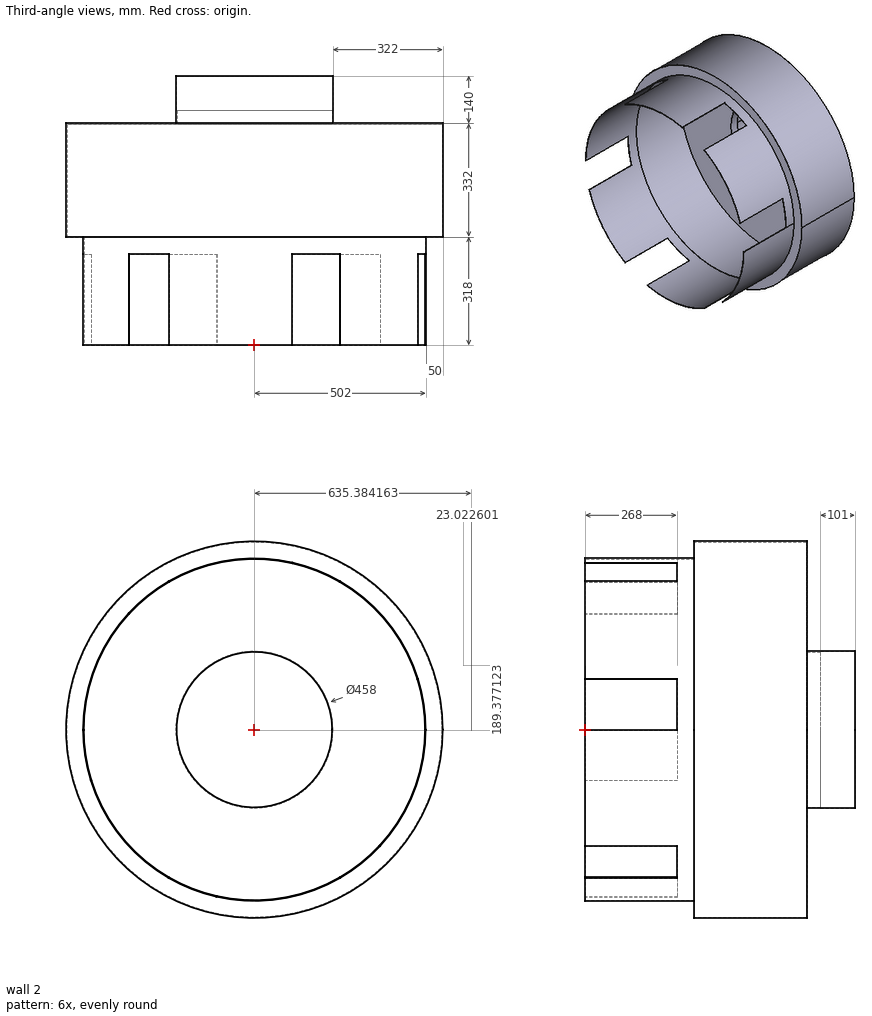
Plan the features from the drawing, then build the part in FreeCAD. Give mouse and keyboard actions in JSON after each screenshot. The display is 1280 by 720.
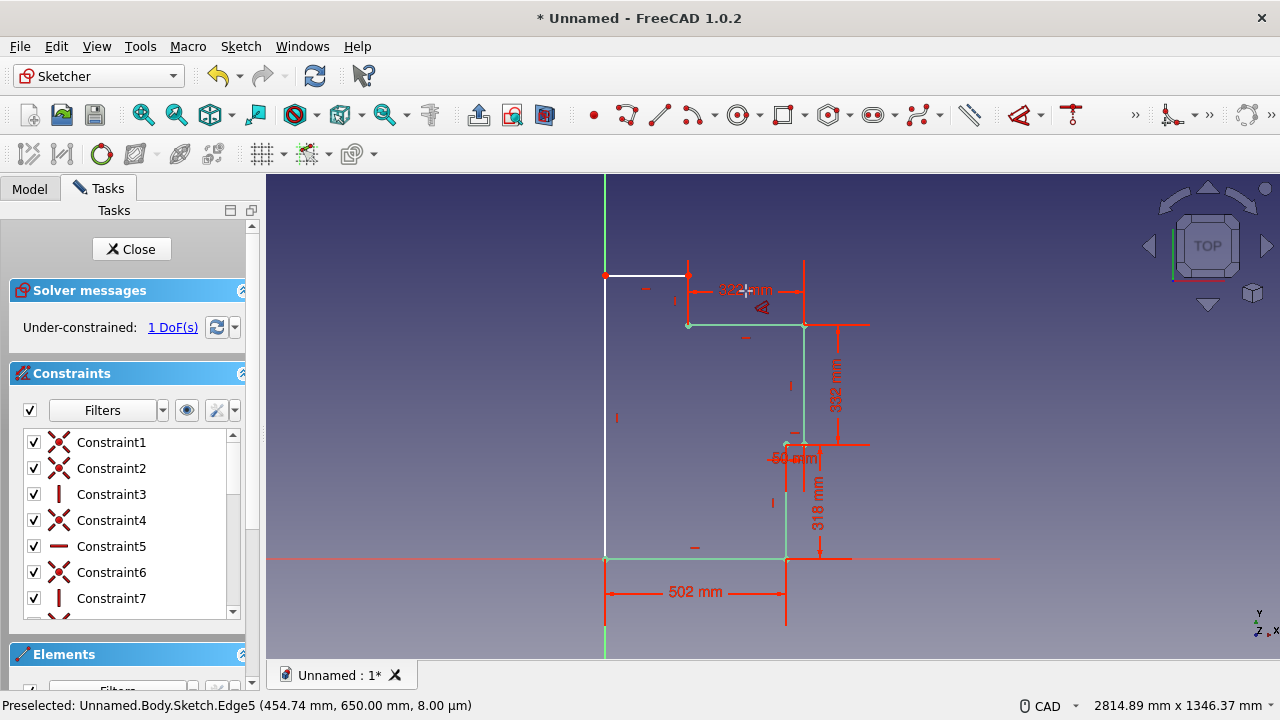
{"action": "left_click", "coordinate": [688, 310]}
{"action": "left_click", "coordinate": [654, 301]}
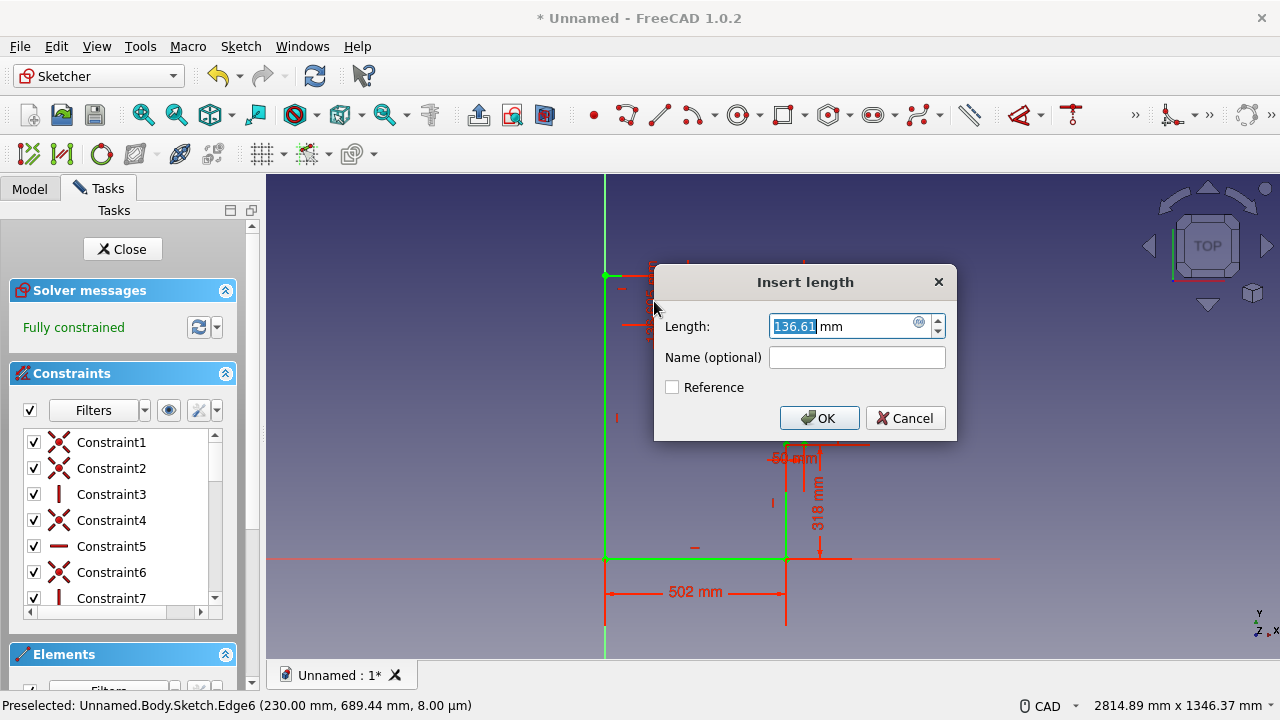
{"action": "type", "text": "140"}
{"action": "key", "text": "Return"}
{"action": "key", "text": "Escape"}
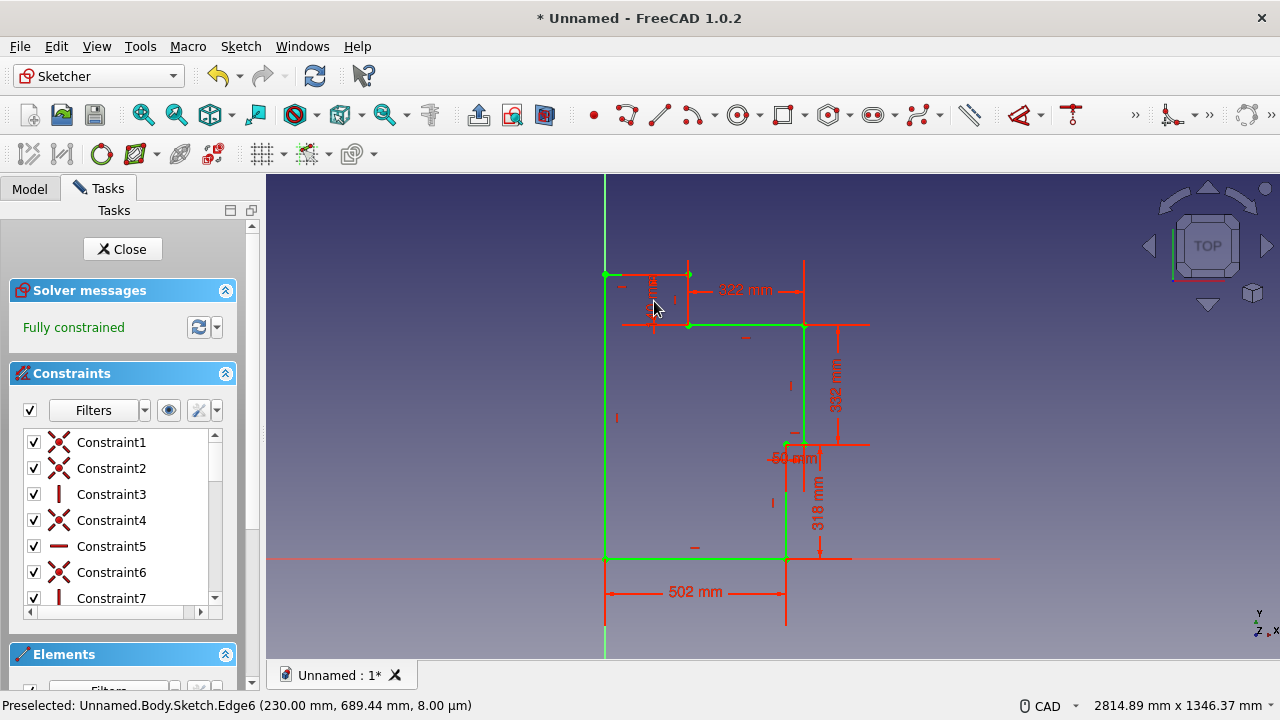
{"action": "left_click", "coordinate": [123, 249]}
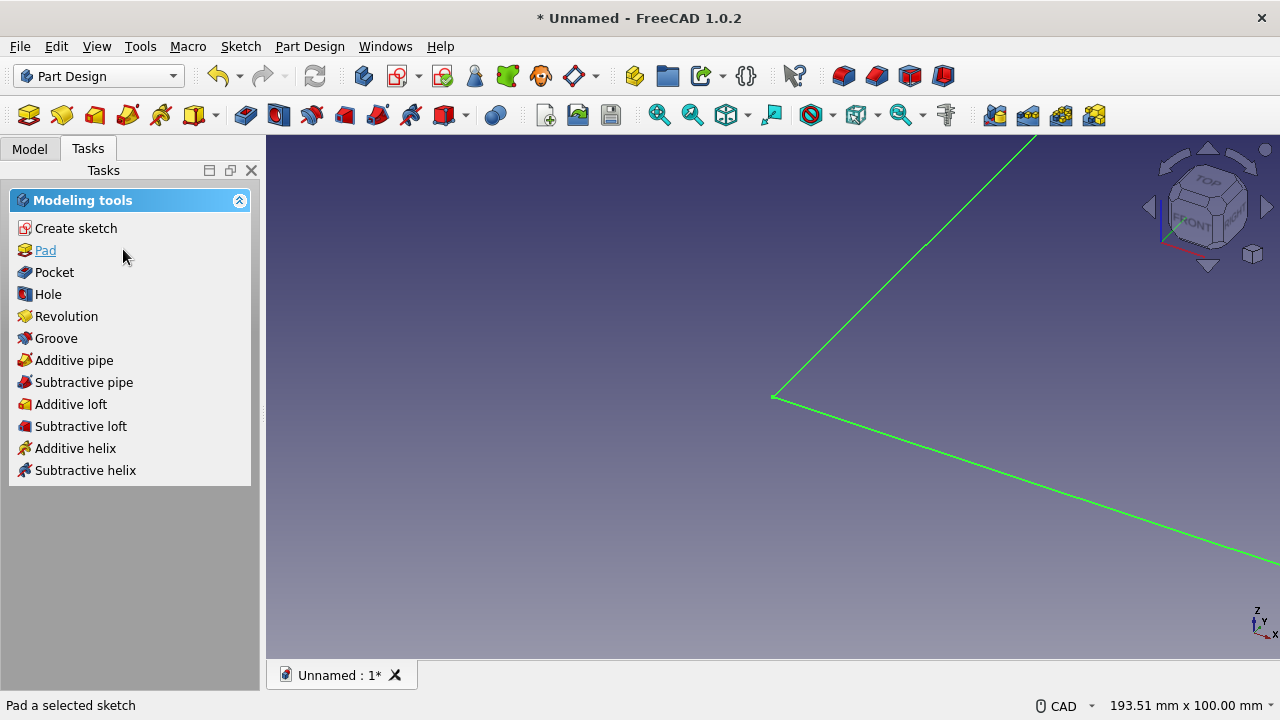
{"action": "left_click", "coordinate": [62, 116]}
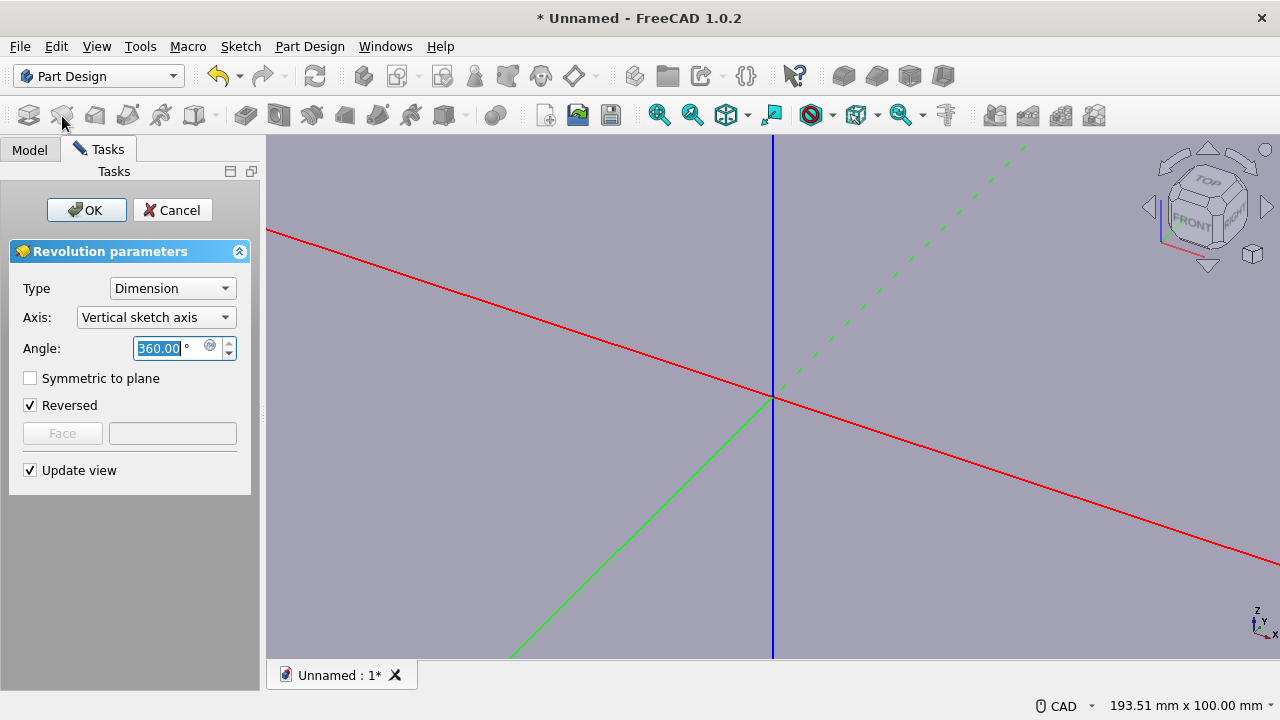
{"action": "left_click", "coordinate": [87, 210]}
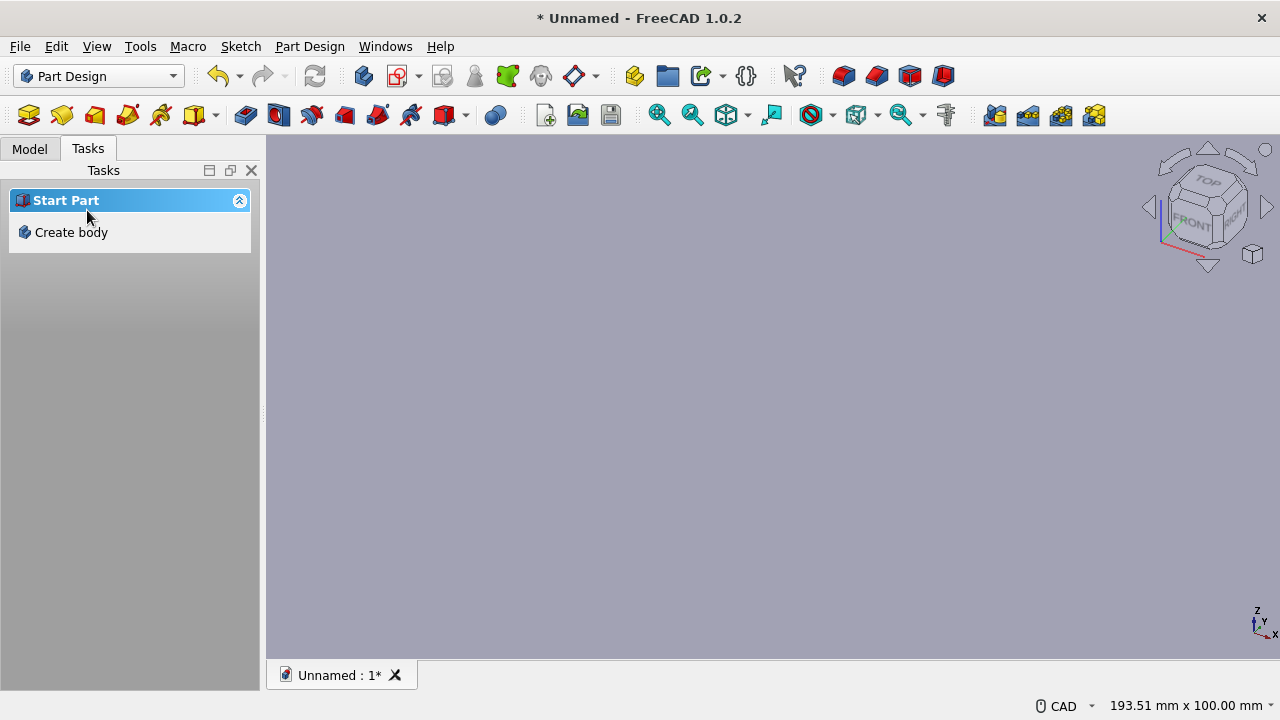
{"action": "left_click", "coordinate": [660, 116]}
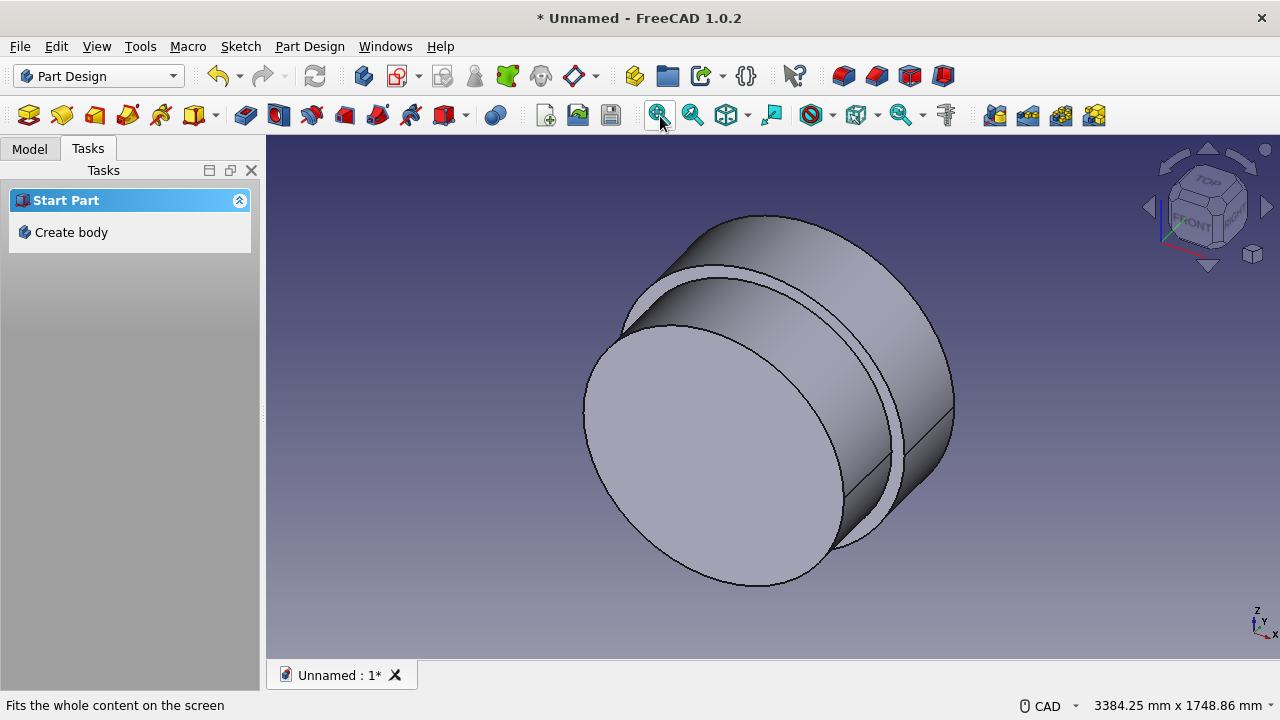
{"action": "left_click", "coordinate": [714, 455]}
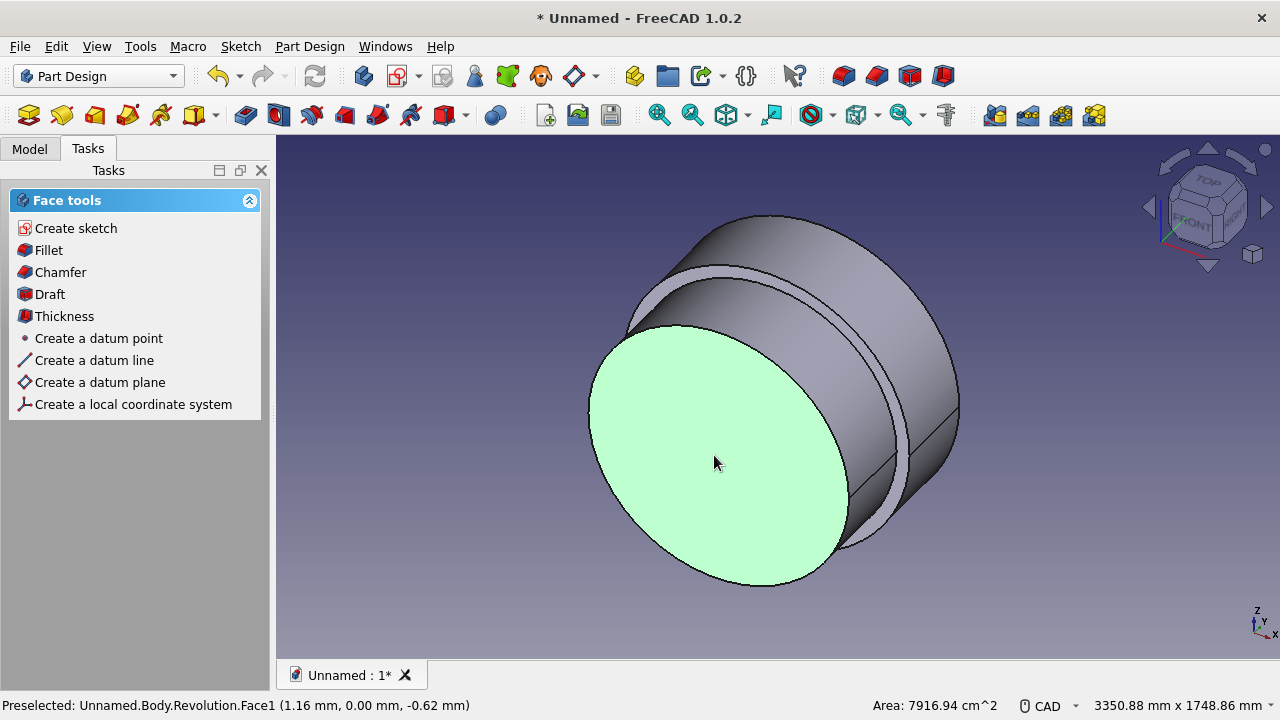
{"action": "left_click", "coordinate": [943, 76]}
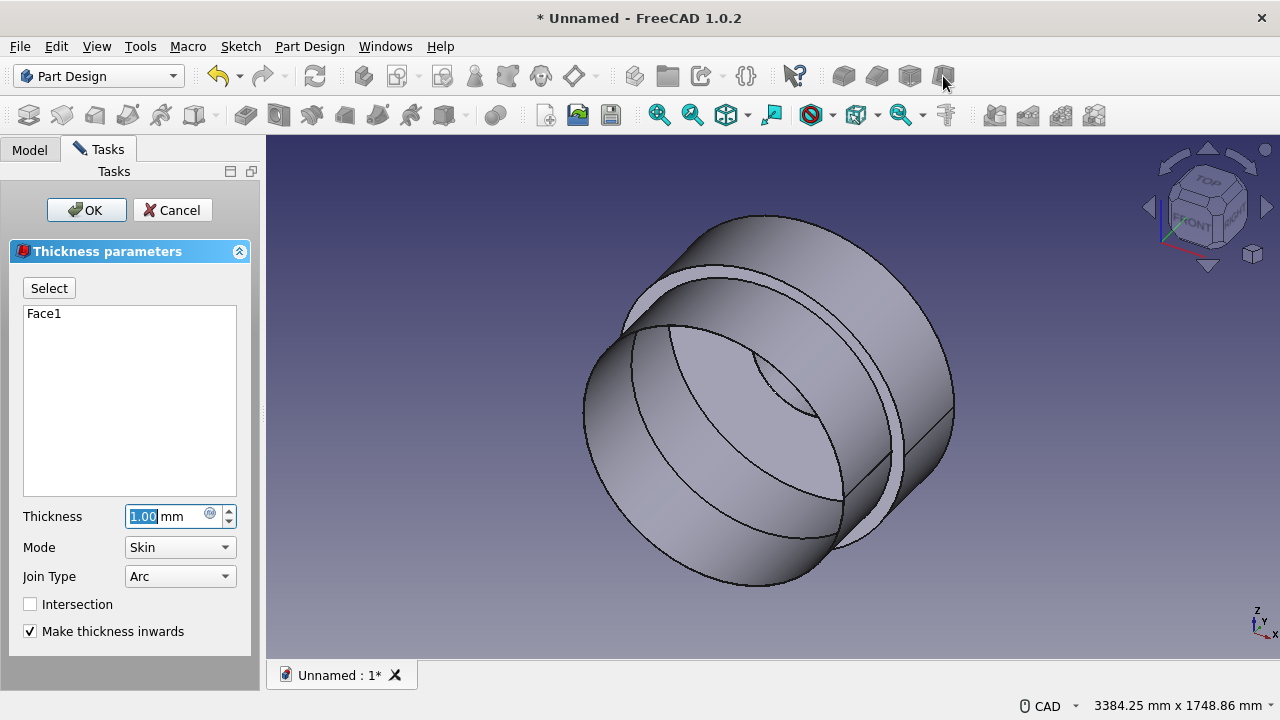
{"action": "type", "text": "2"}
{"action": "key", "text": "Tab"}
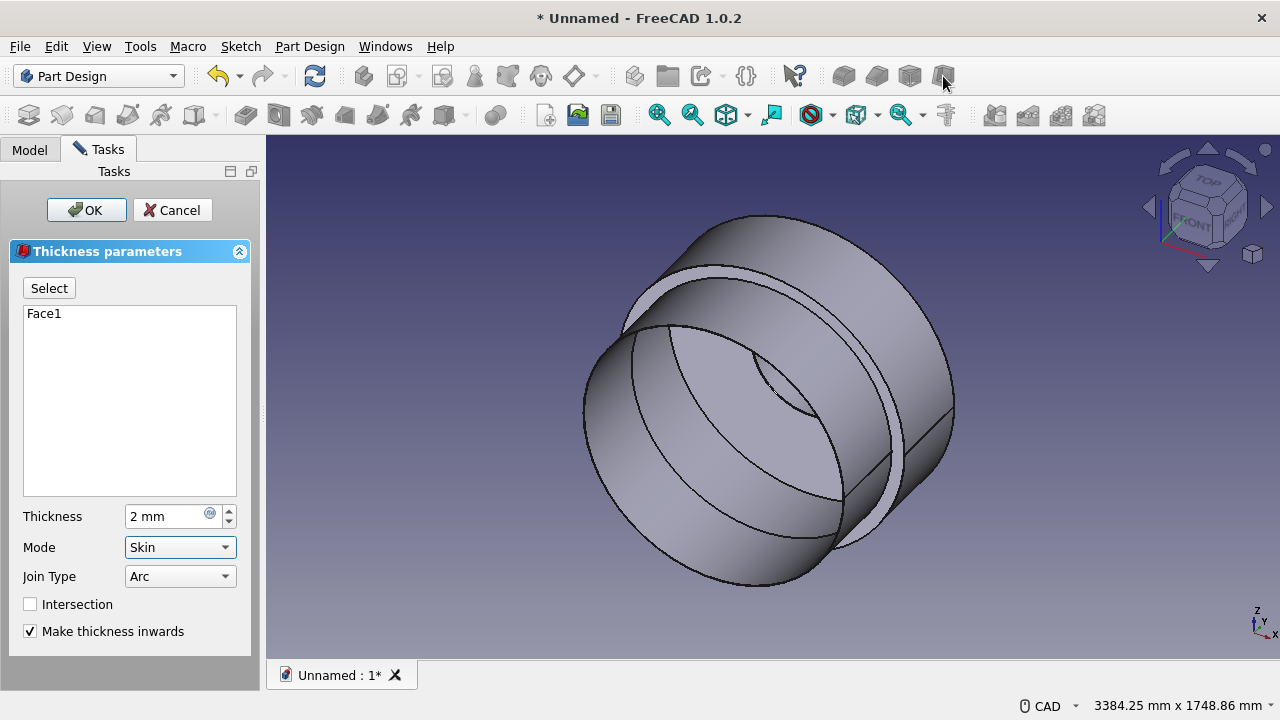
{"action": "left_click", "coordinate": [181, 576]}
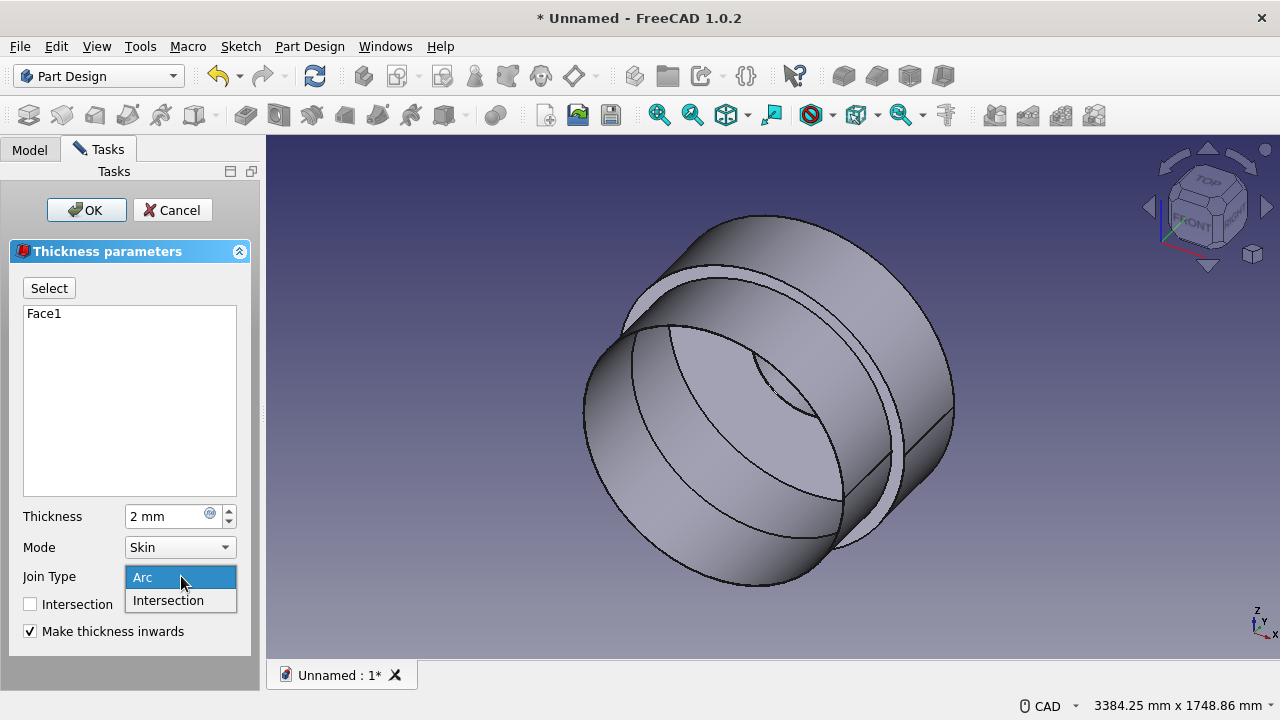
{"action": "left_click", "coordinate": [179, 600]}